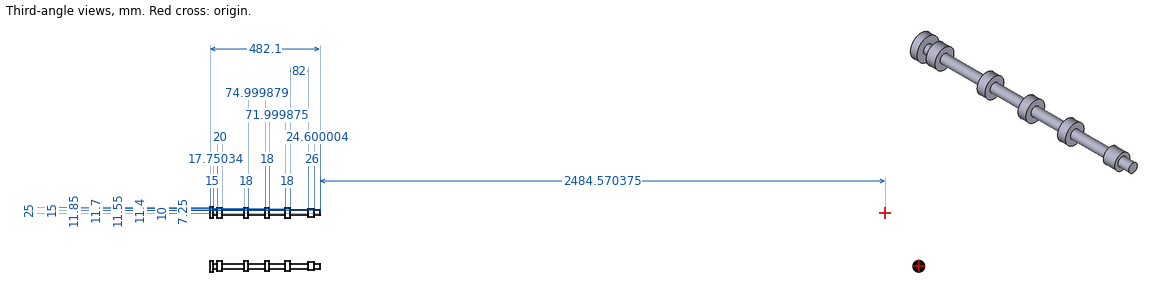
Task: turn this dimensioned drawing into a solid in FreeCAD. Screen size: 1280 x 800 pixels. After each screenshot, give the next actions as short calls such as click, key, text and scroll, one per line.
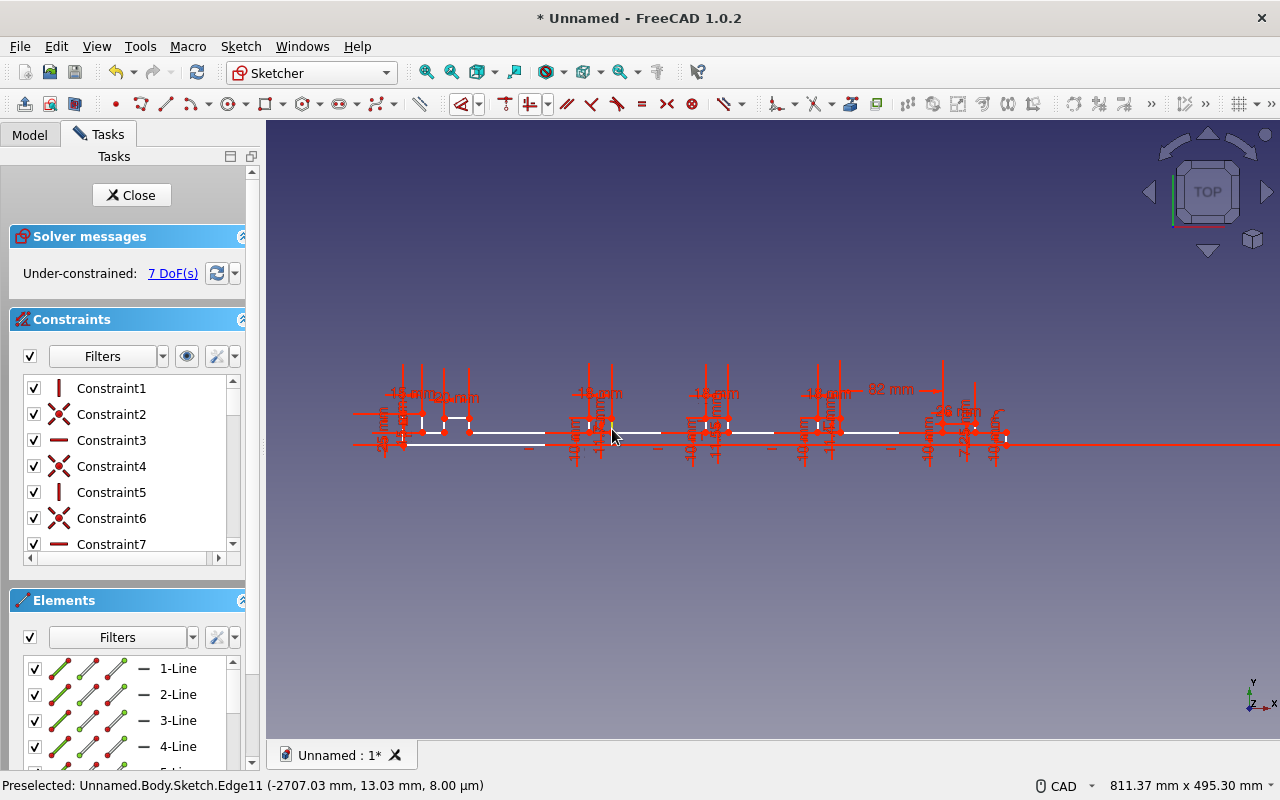
scroll(469, 428, up, 6)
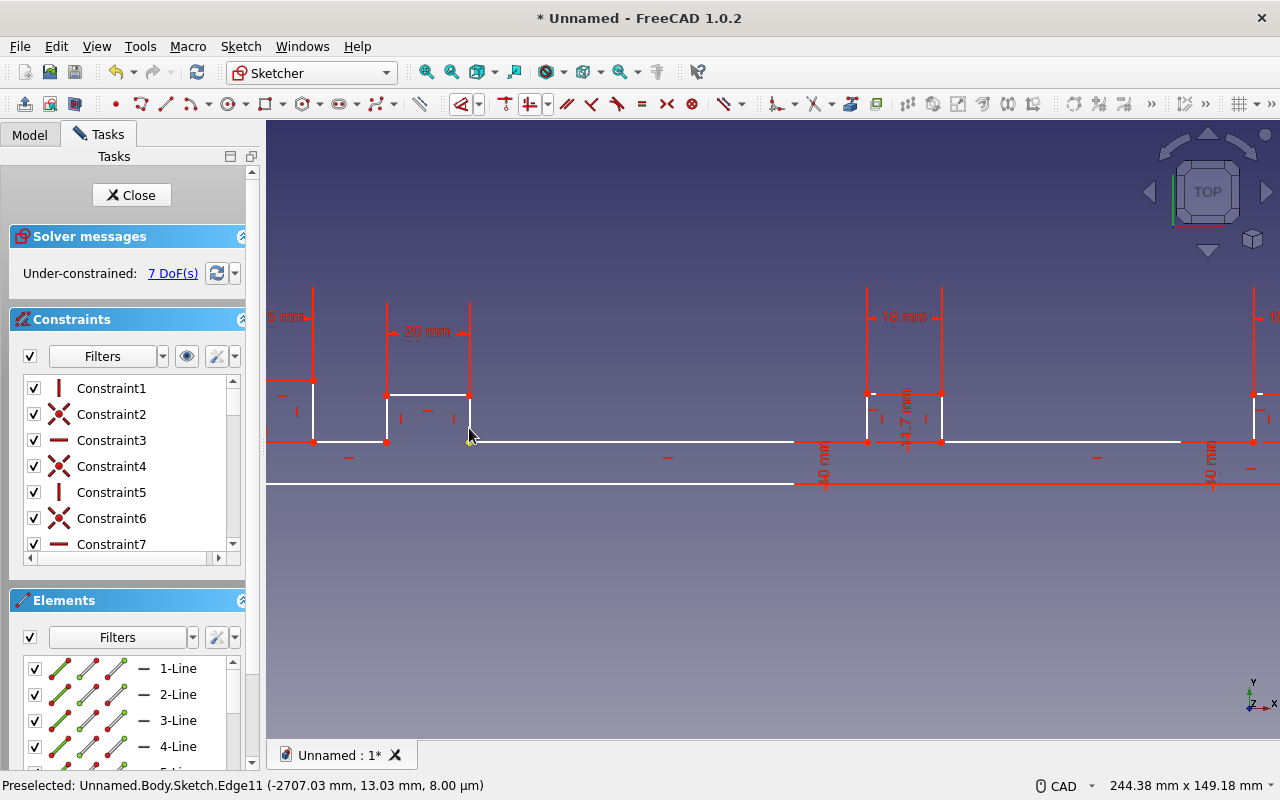
click(470, 428)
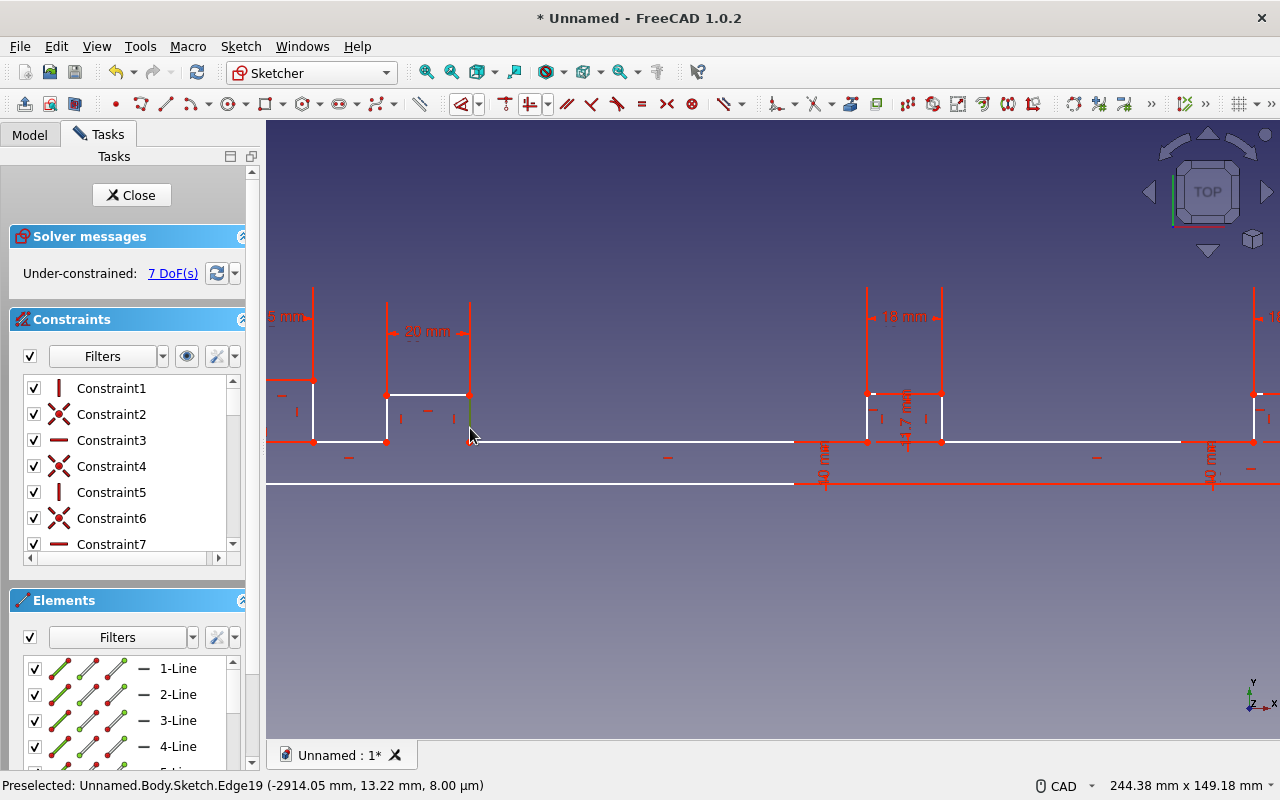
click(478, 104)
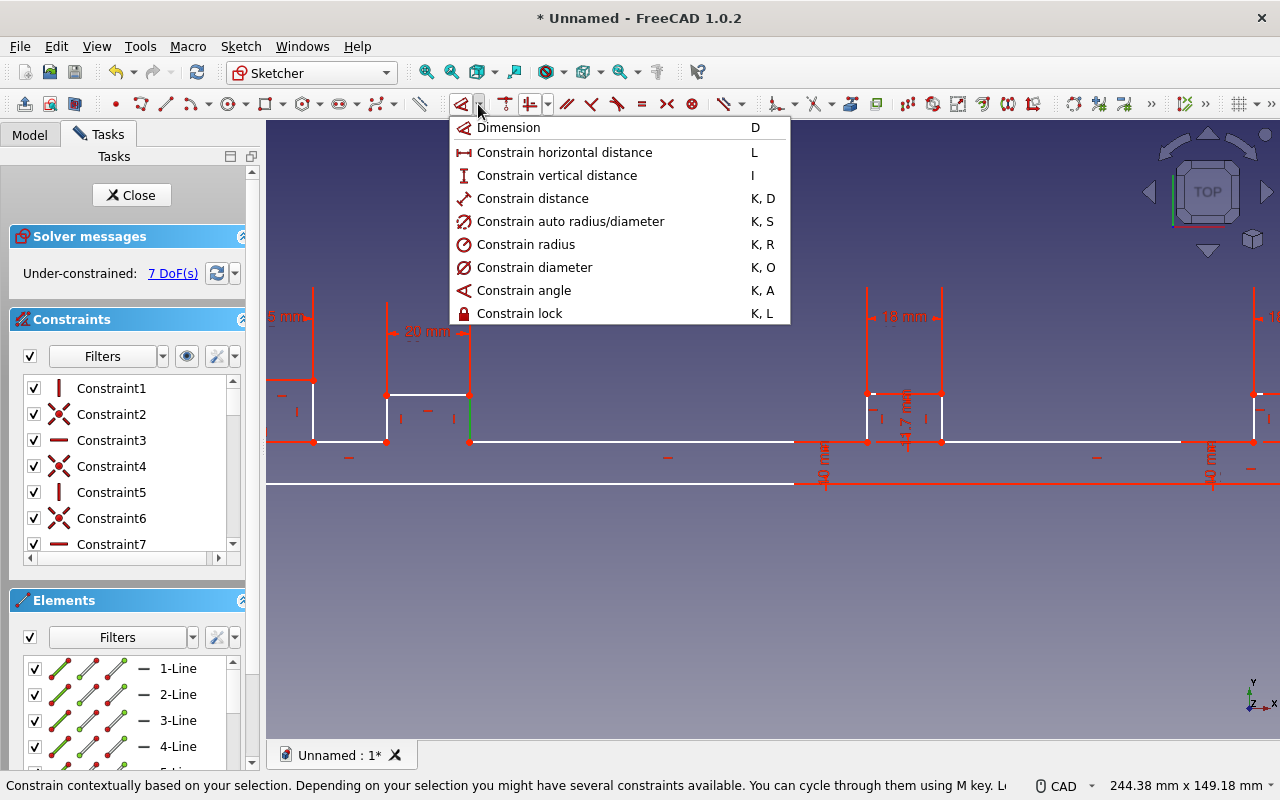
click(620, 176)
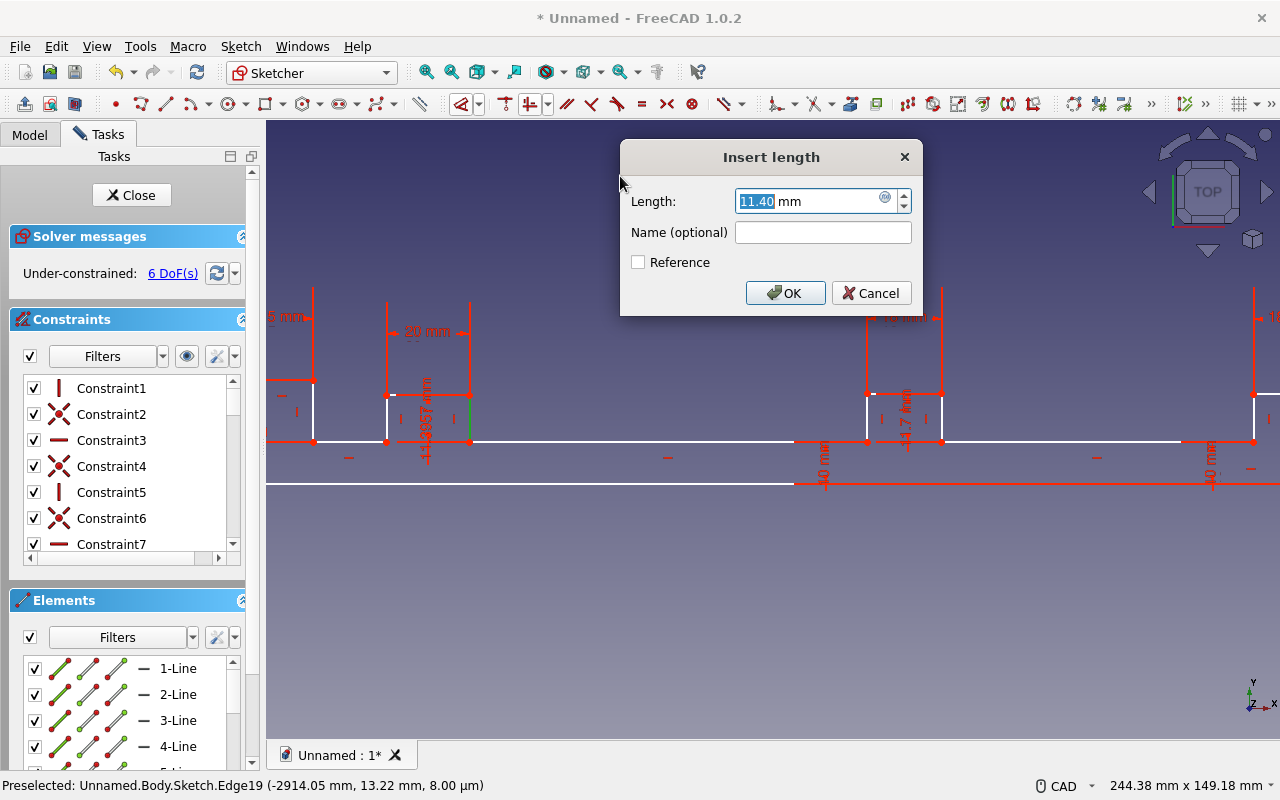
text(11.85)
key(Return)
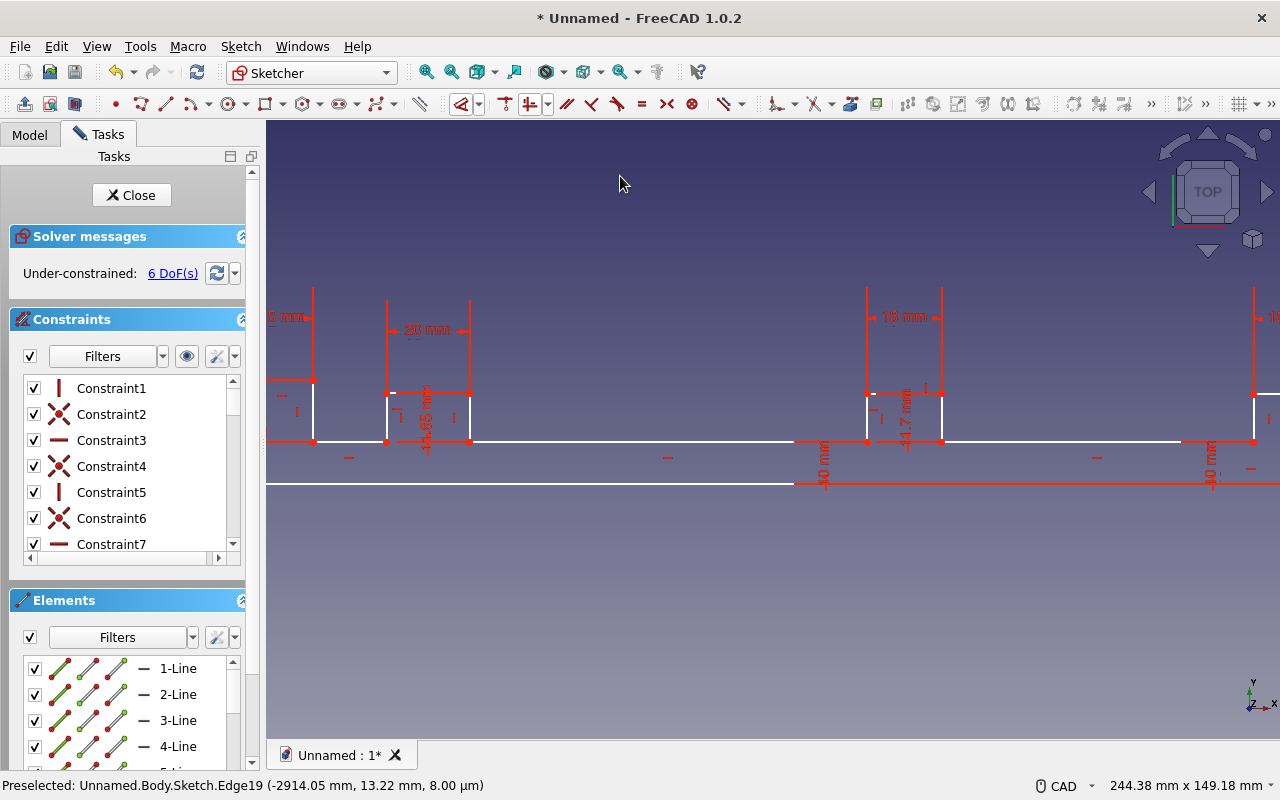
click(852, 484)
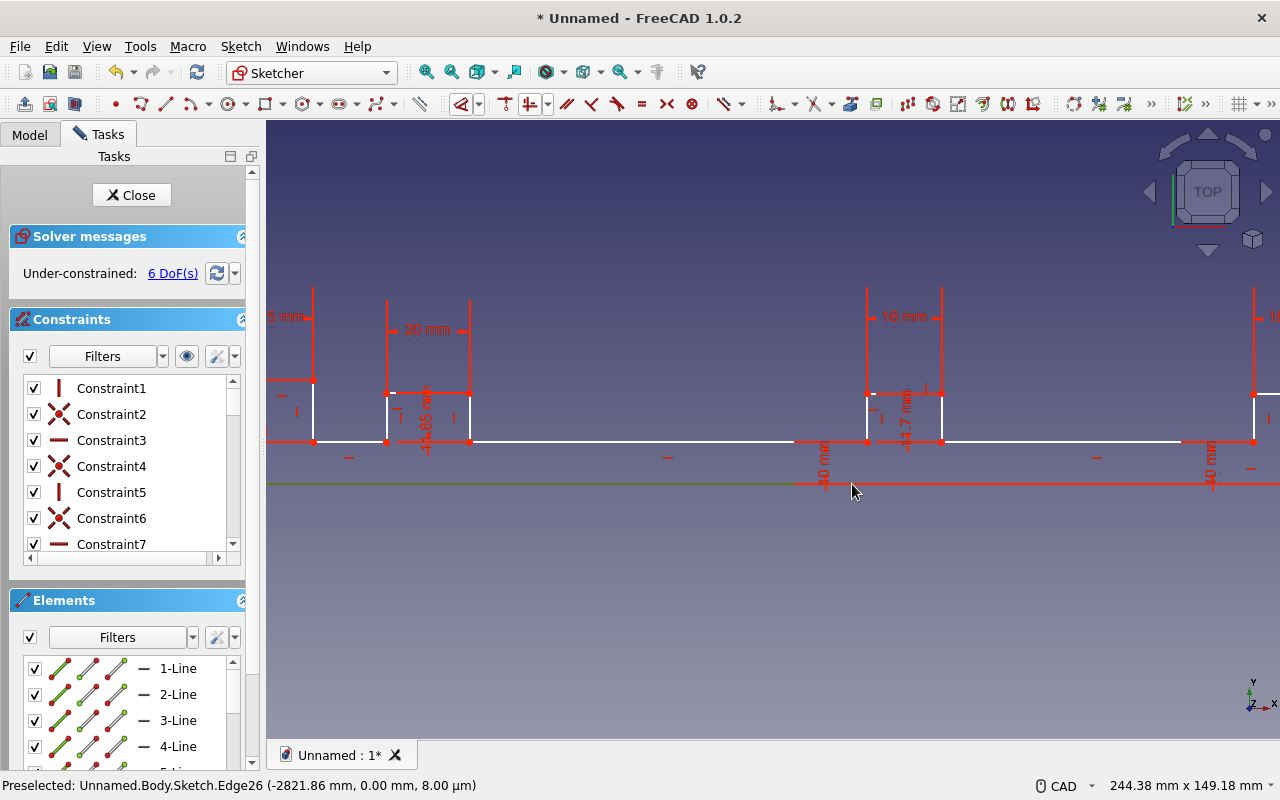
key(l)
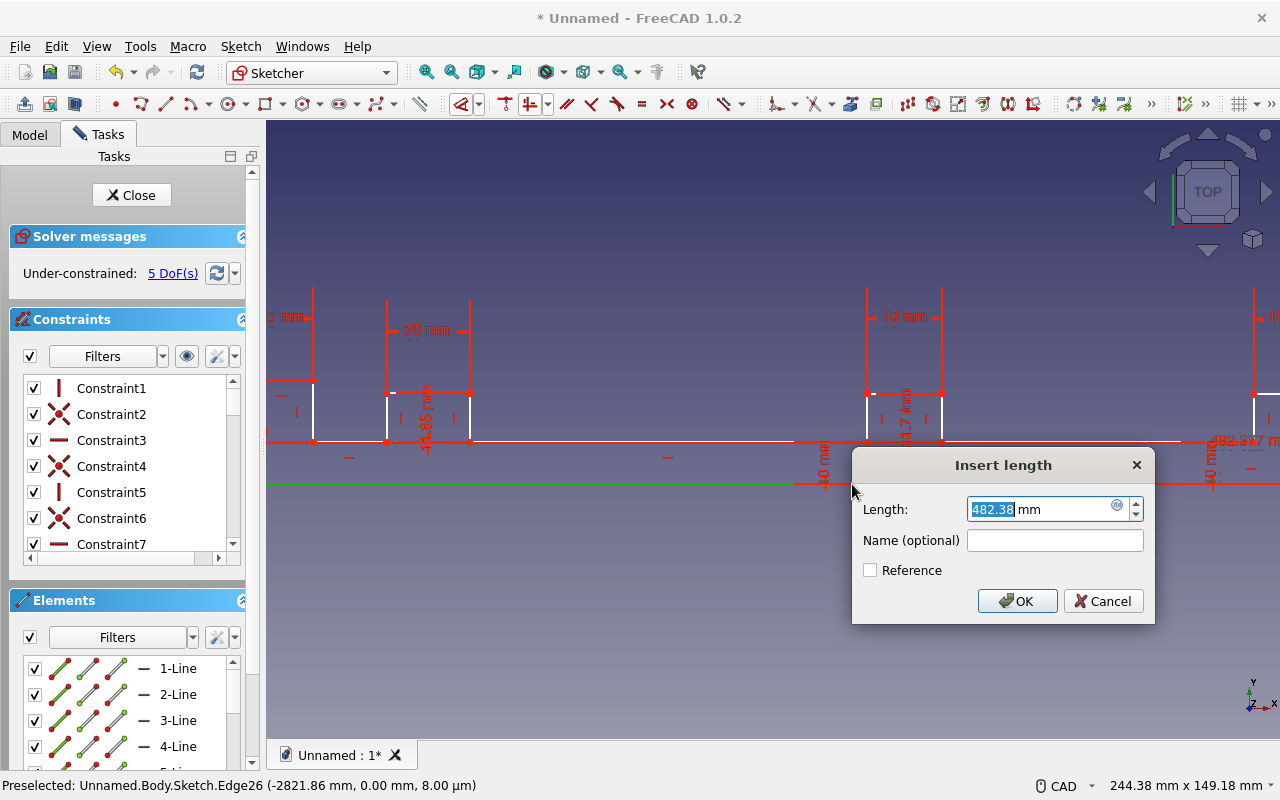
text(482.1)
key(Return)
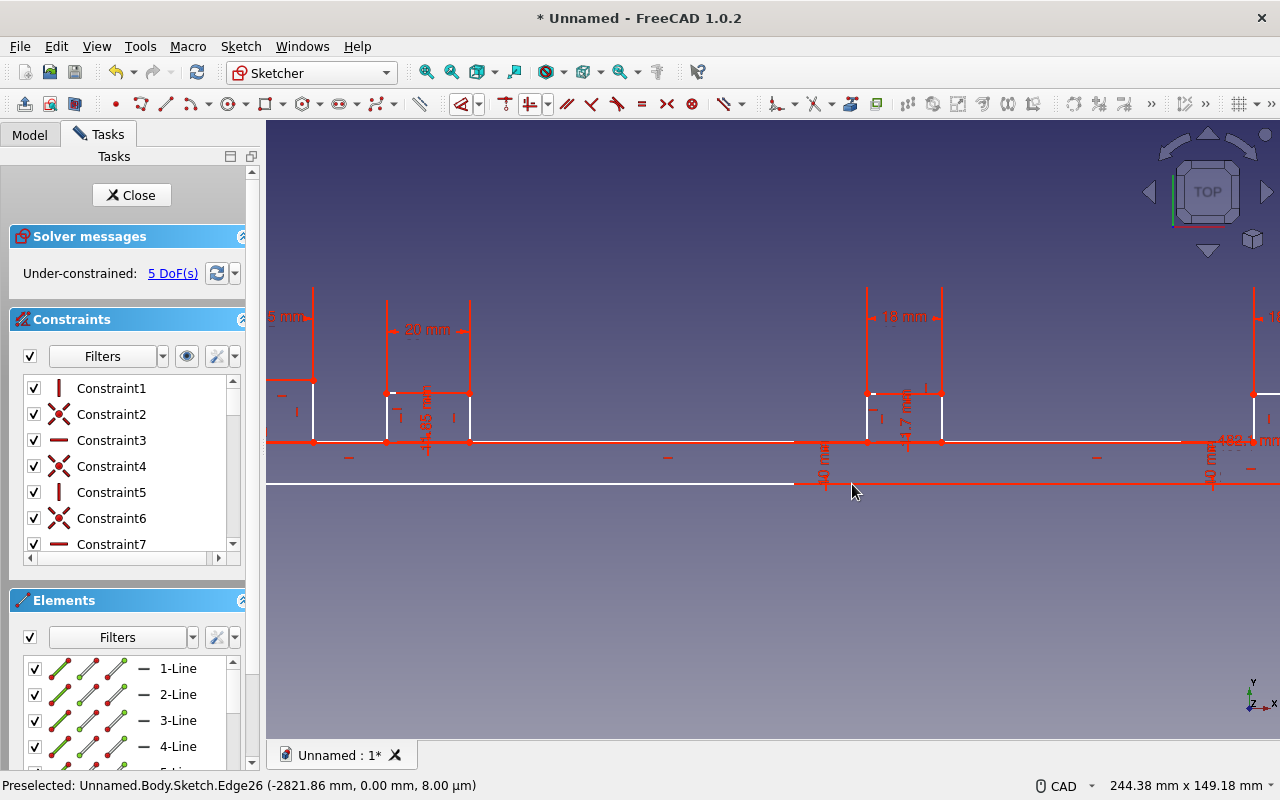
click(365, 442)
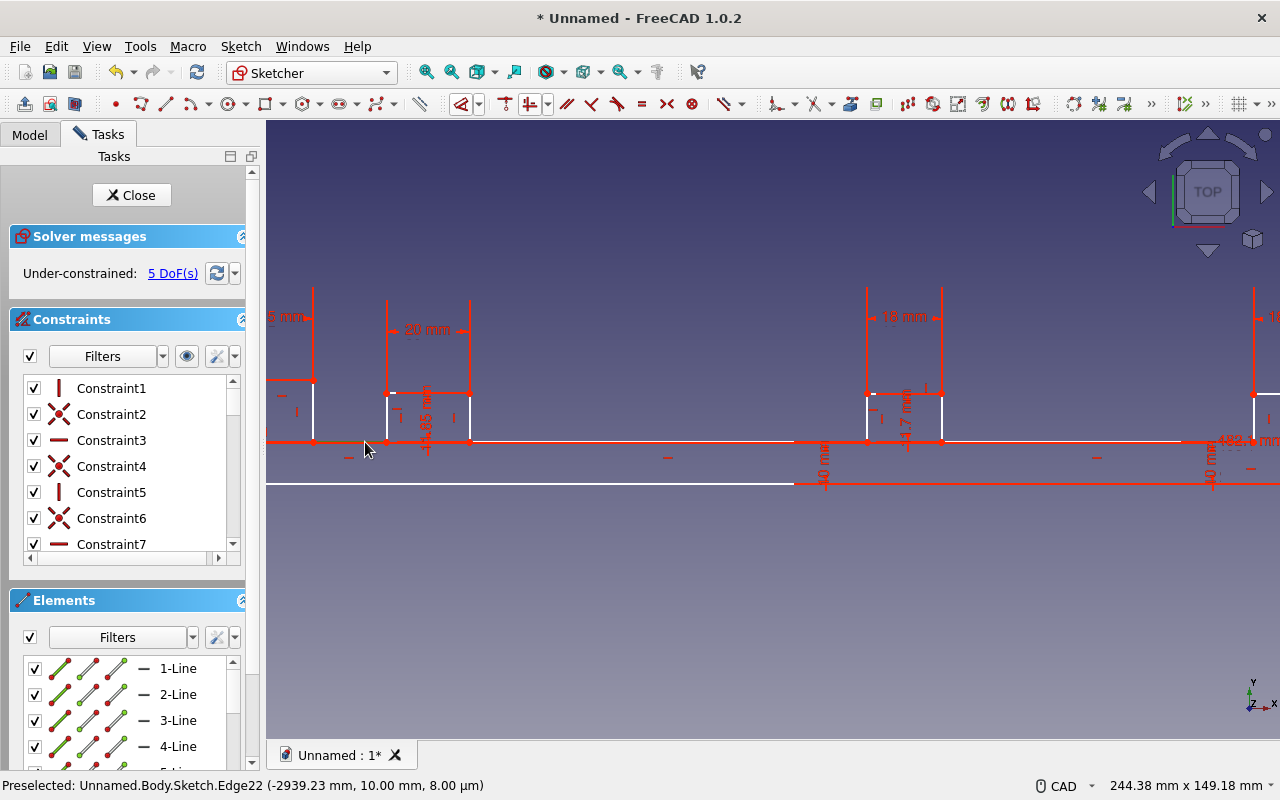
click(478, 104)